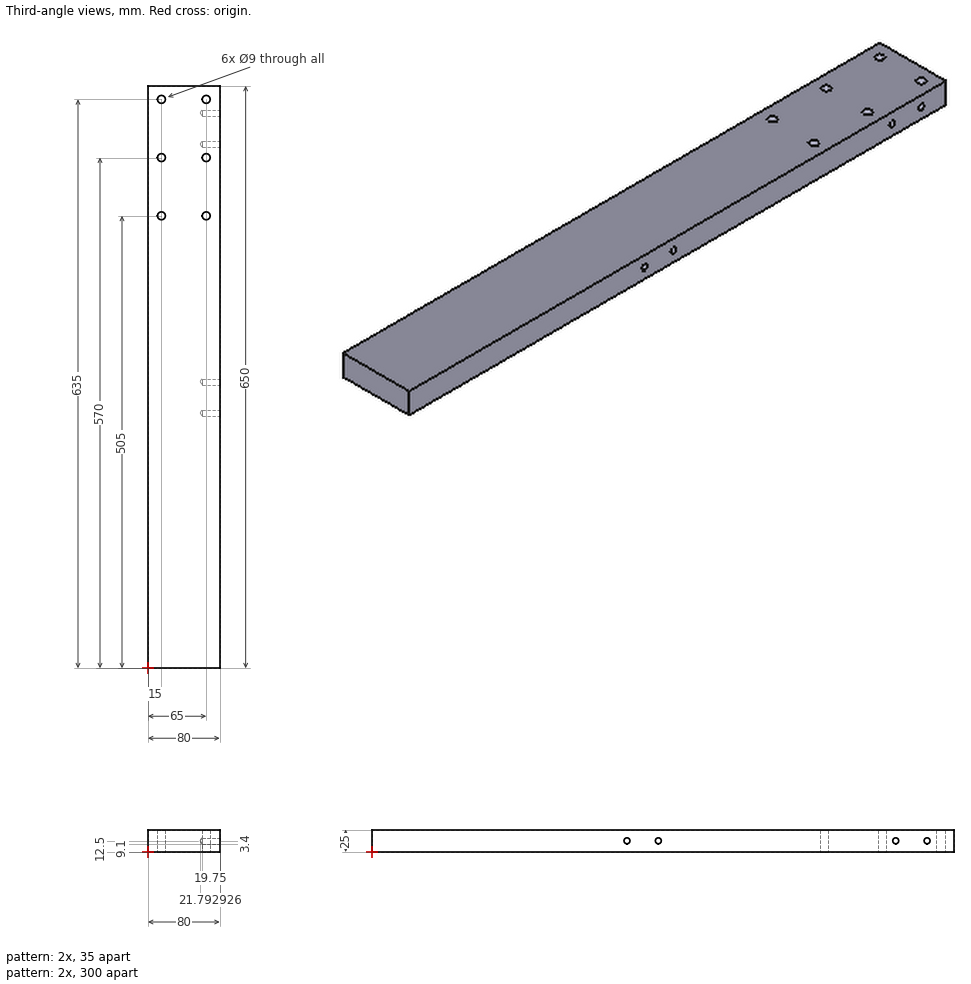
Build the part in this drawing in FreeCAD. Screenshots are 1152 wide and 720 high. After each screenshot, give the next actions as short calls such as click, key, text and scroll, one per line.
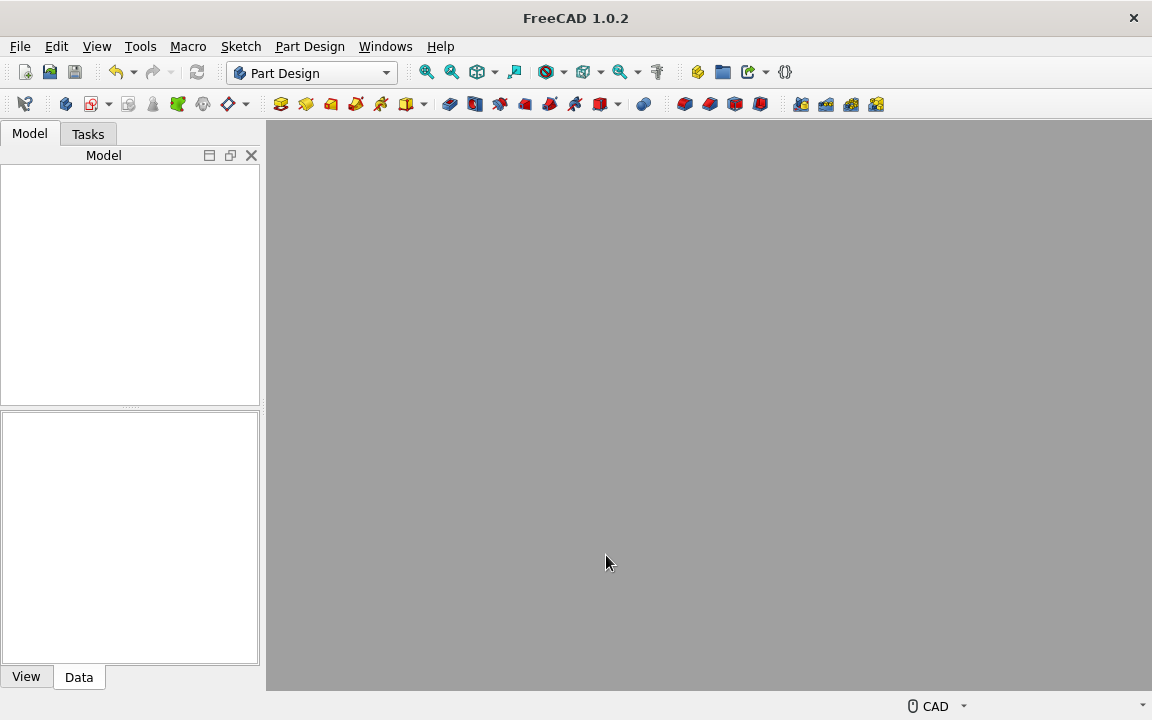
key(ctrl+n)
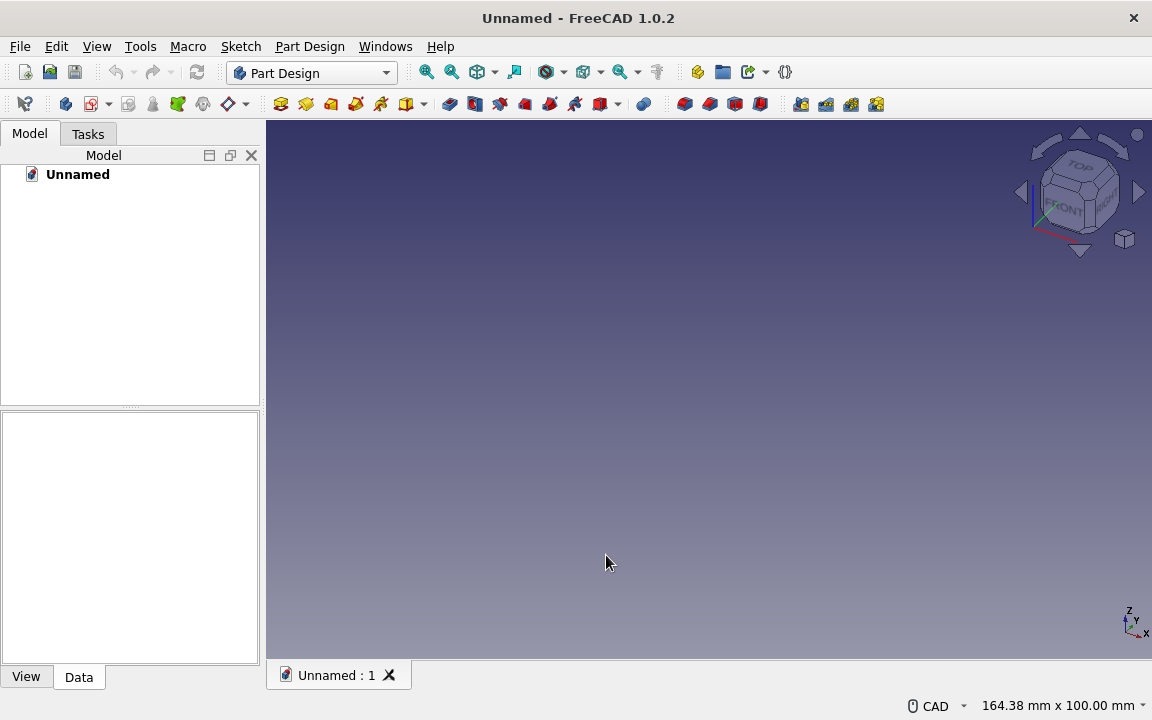
click(90, 104)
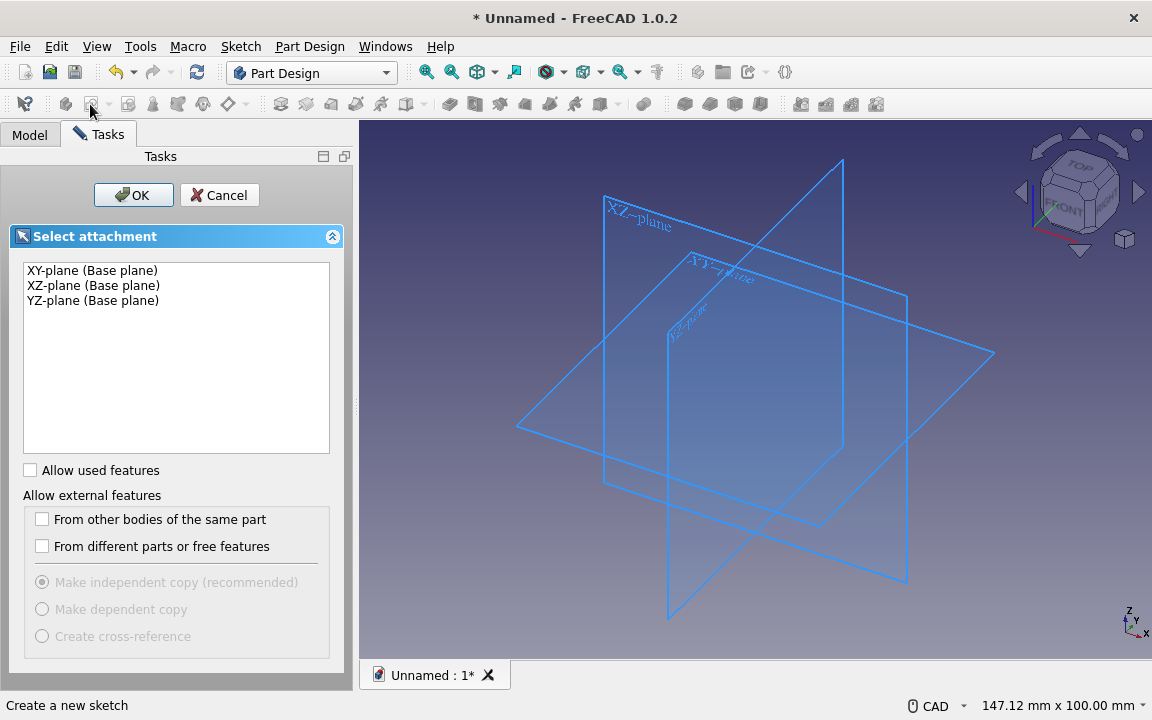
click(84, 270)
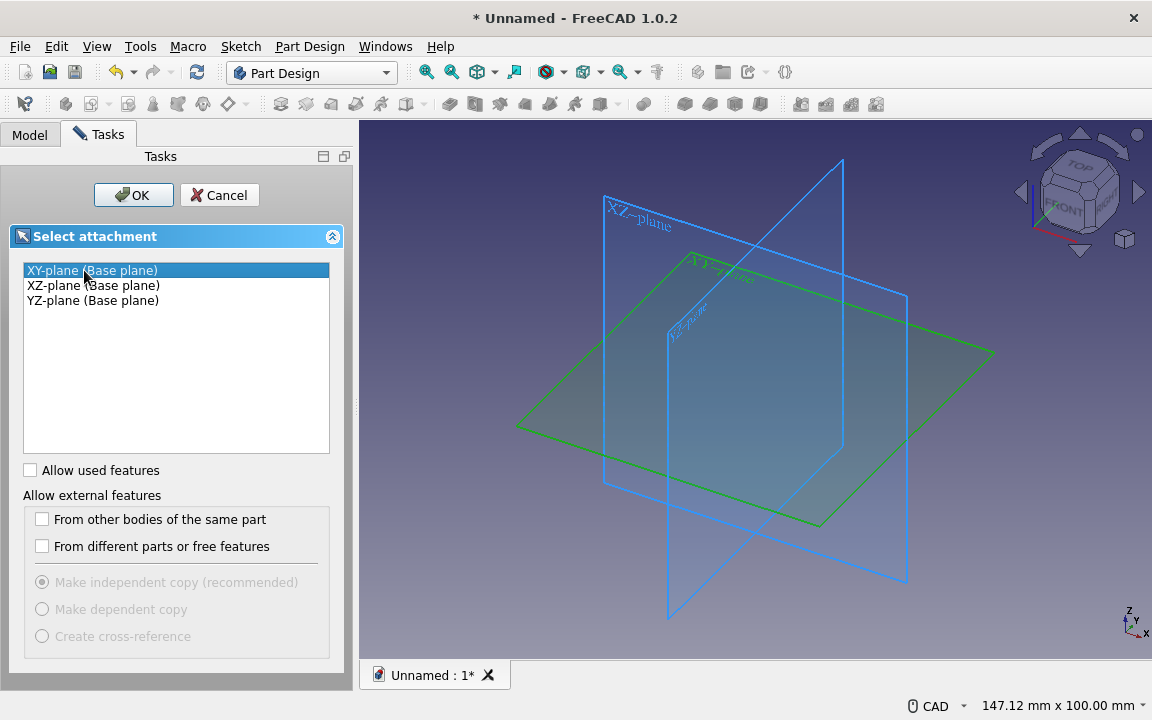
click(134, 195)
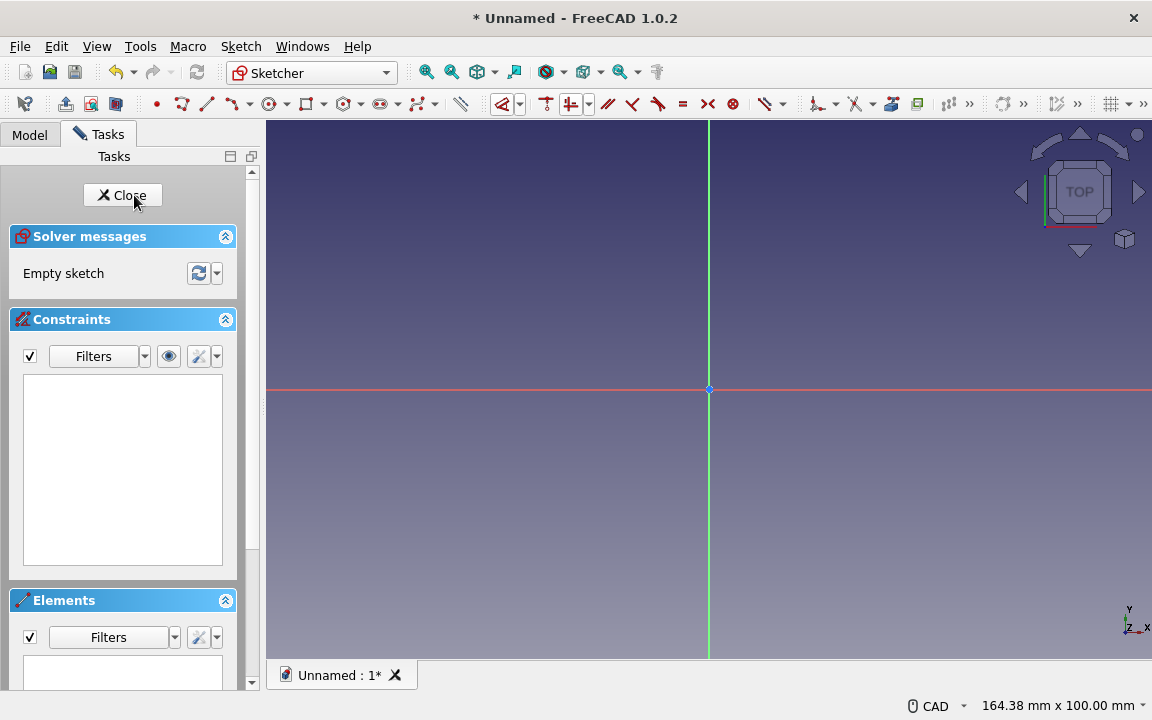
scroll(612, 564, down, 12)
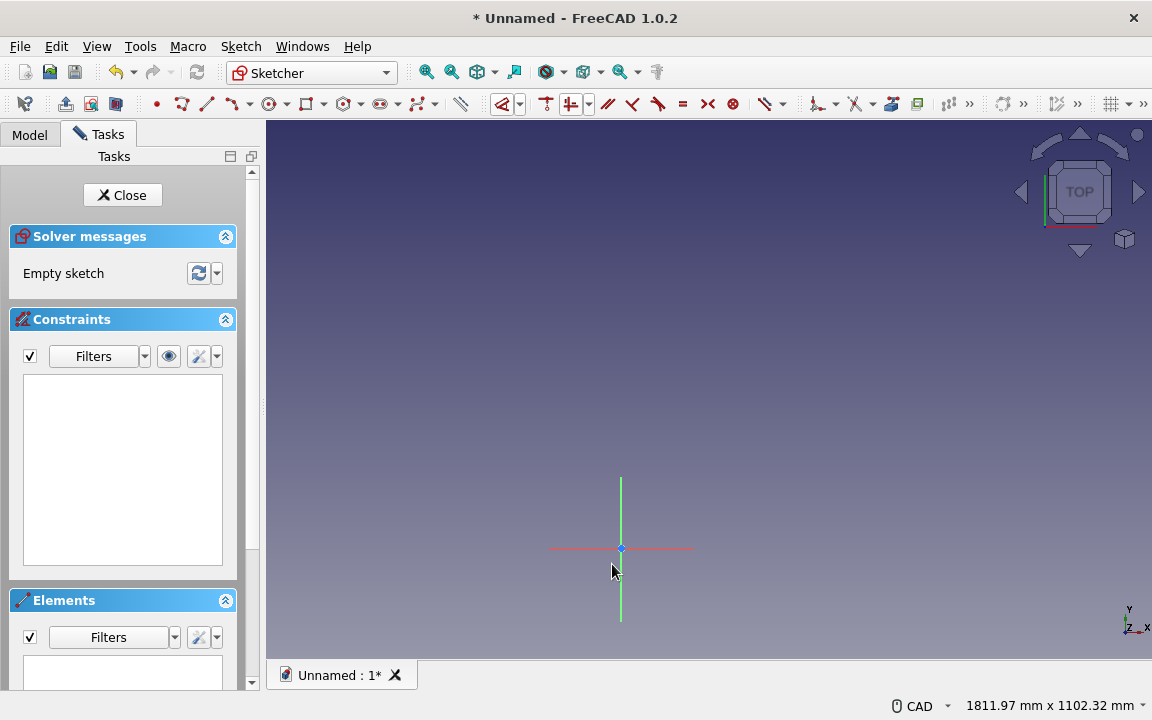
click(306, 104)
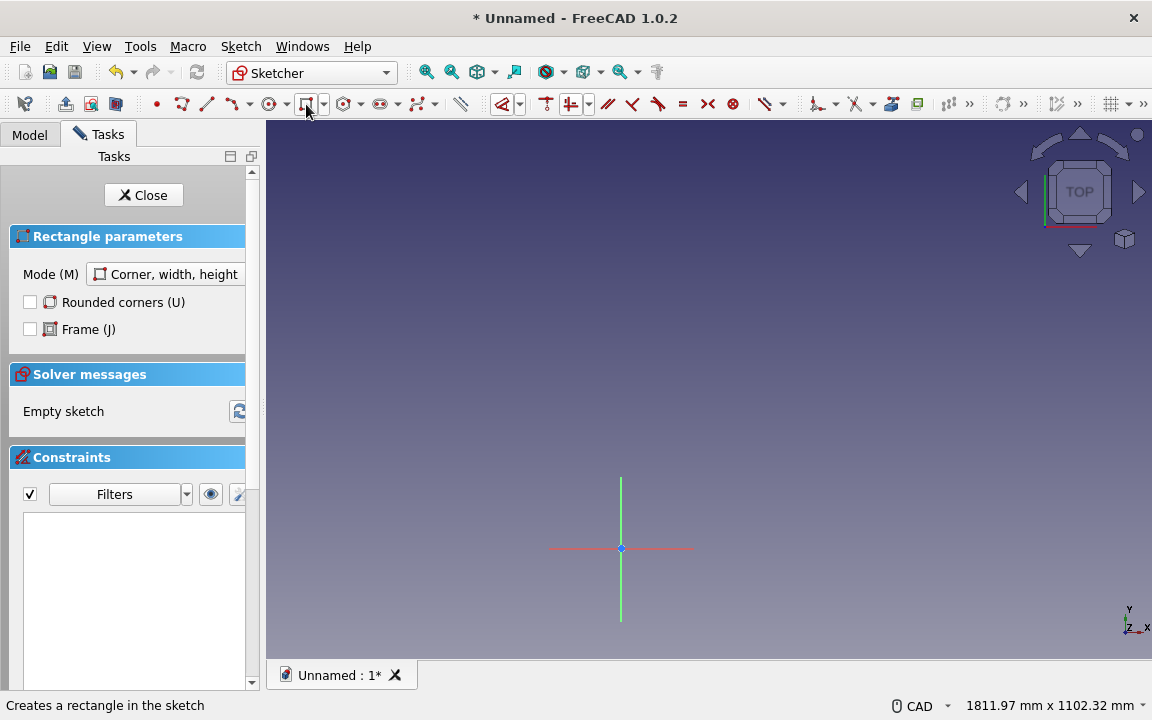
click(621, 549)
move(660, 231)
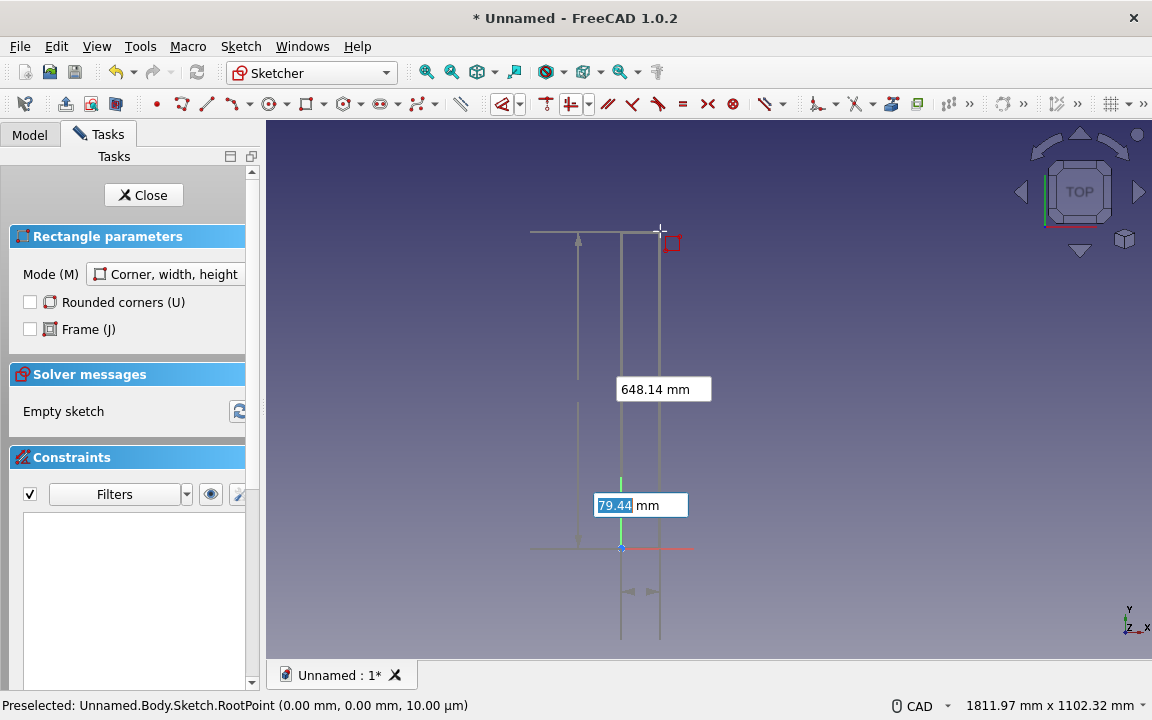
text(80)
key(Tab)
text(650)
key(Return)
key(Escape)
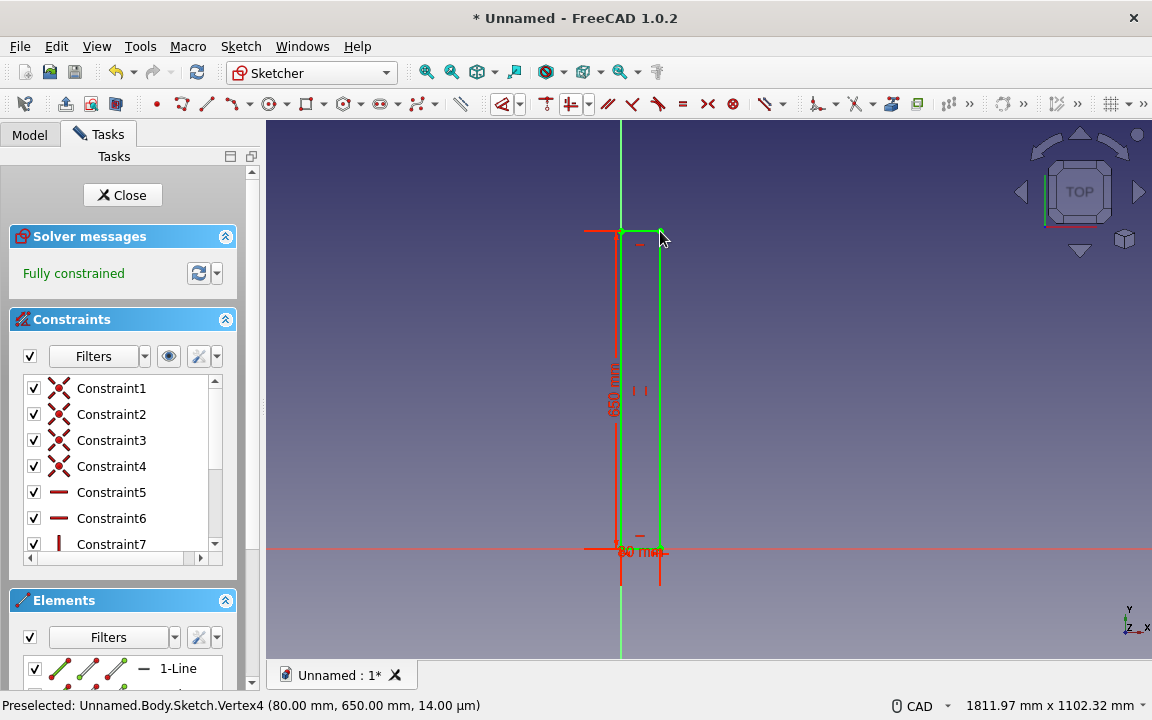
click(123, 195)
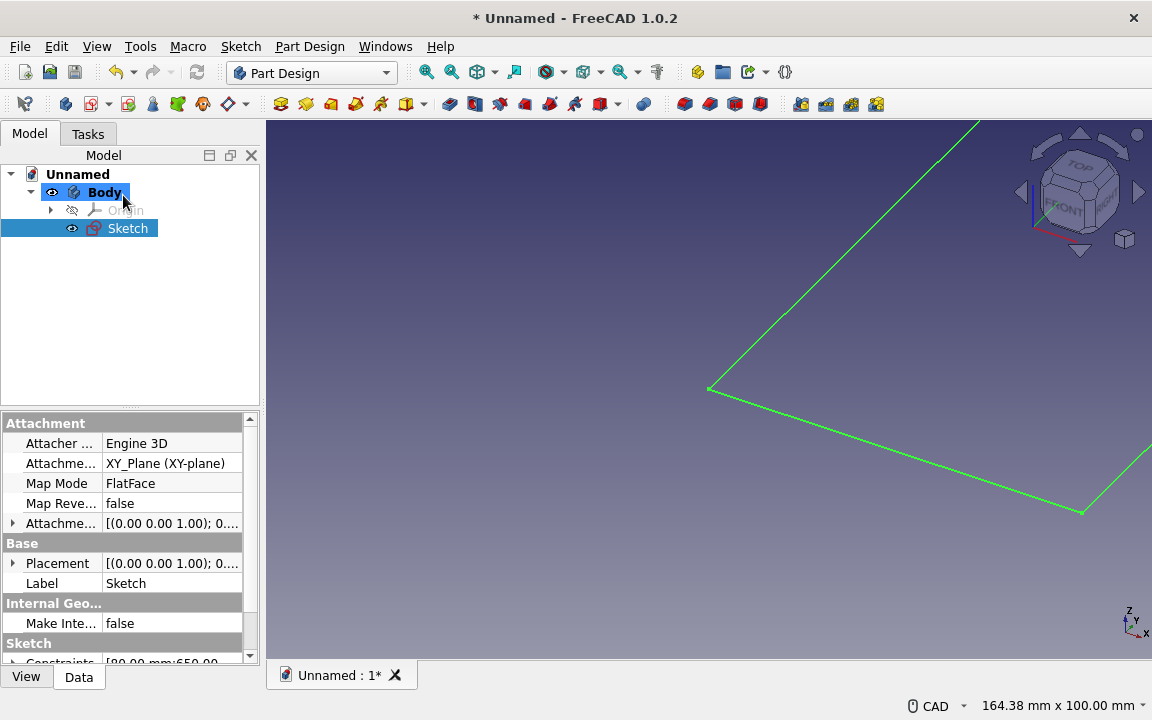
click(281, 104)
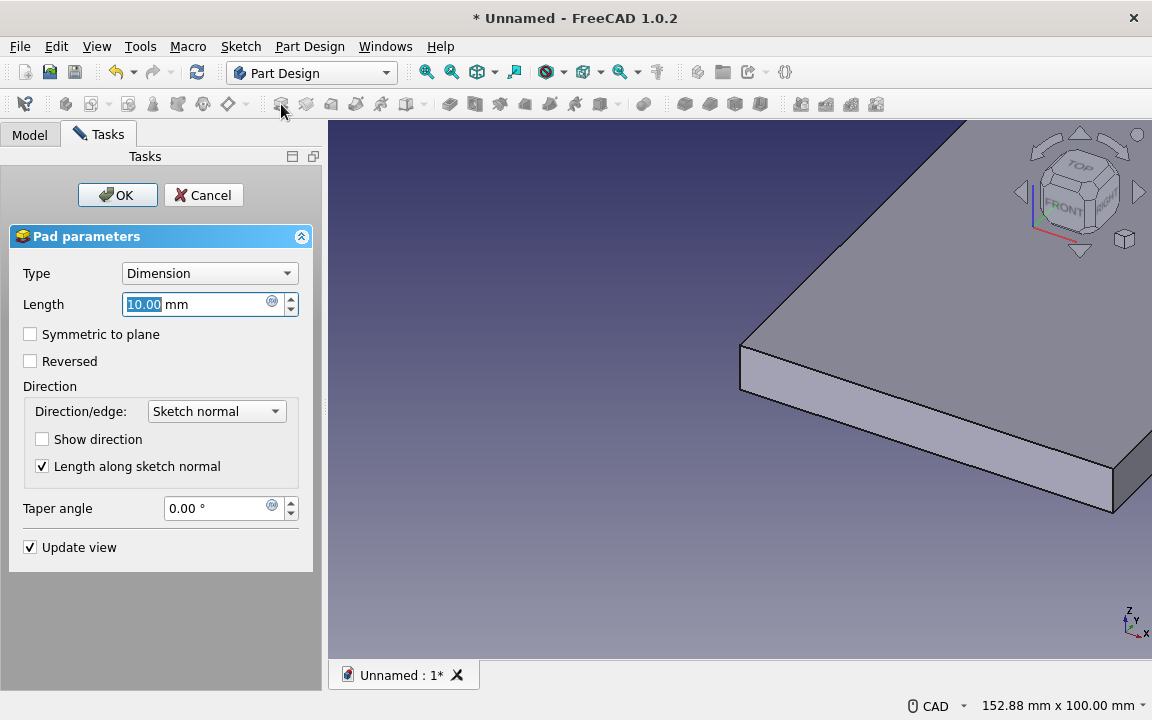
text(25)
key(Tab)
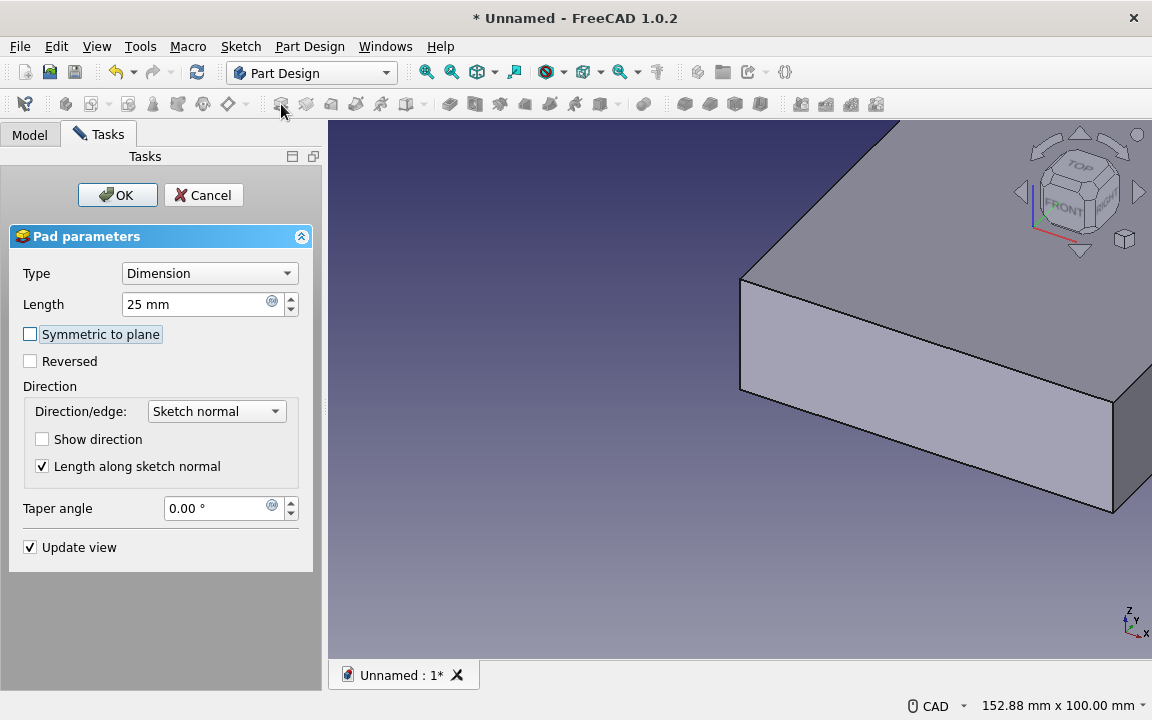
click(118, 195)